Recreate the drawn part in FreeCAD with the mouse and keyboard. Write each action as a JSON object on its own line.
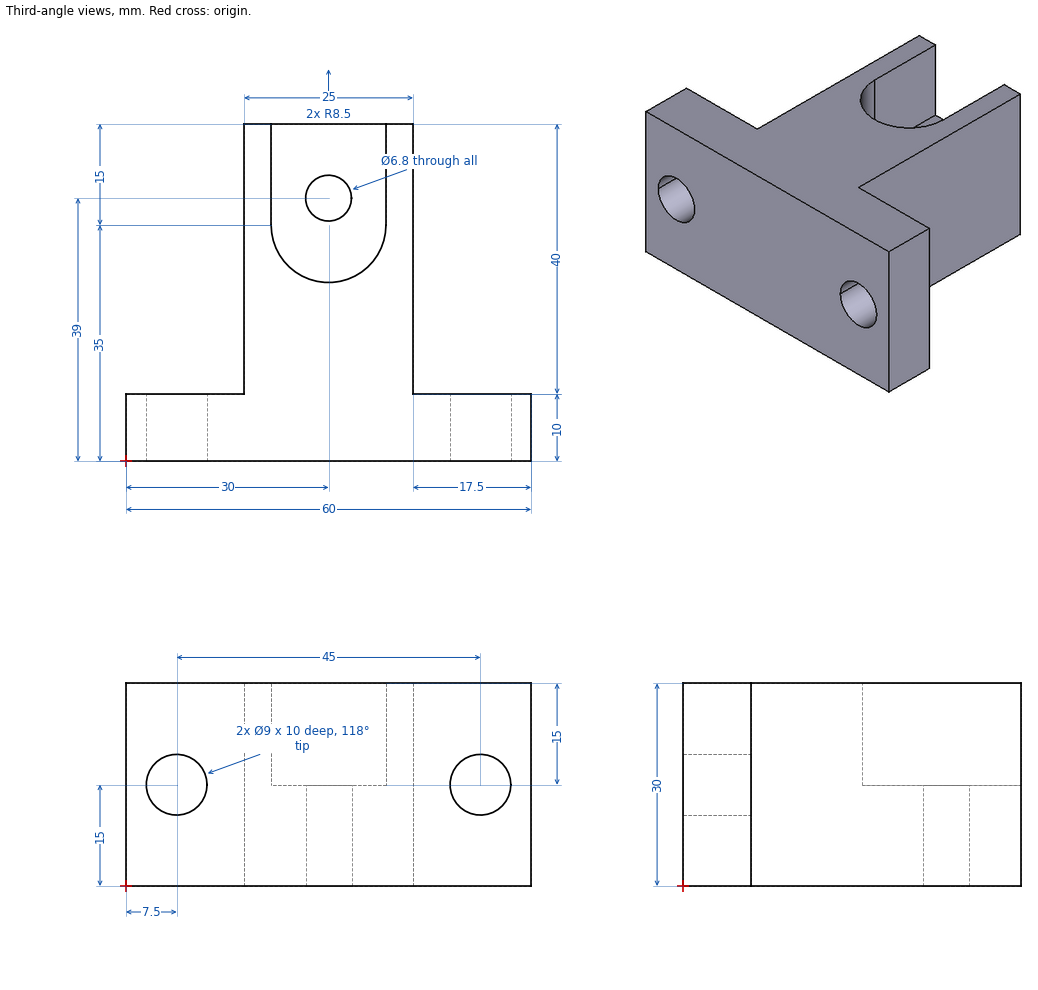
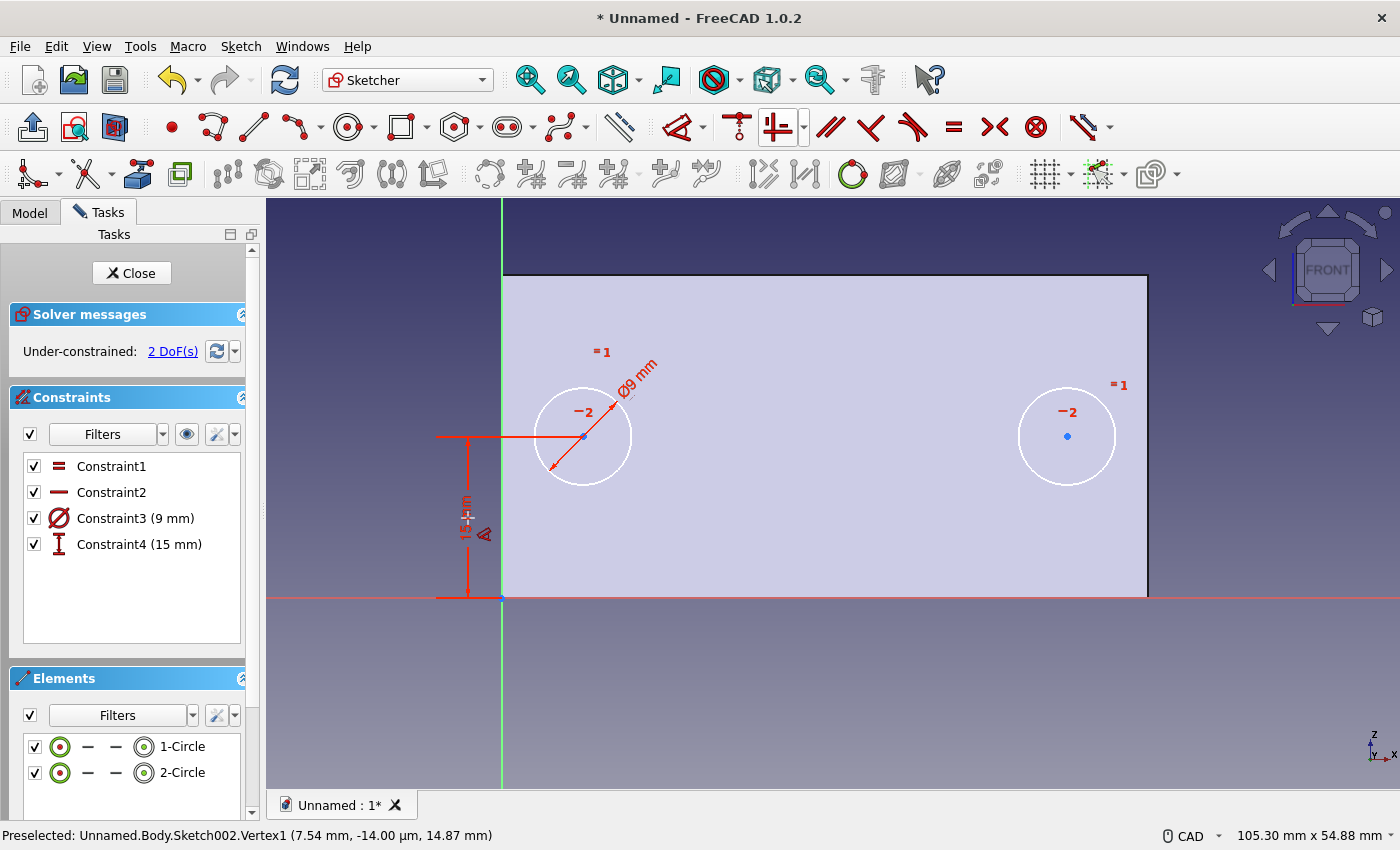
{"action": "left_click", "coordinate": [583, 437]}
{"action": "left_click", "coordinate": [542, 632]}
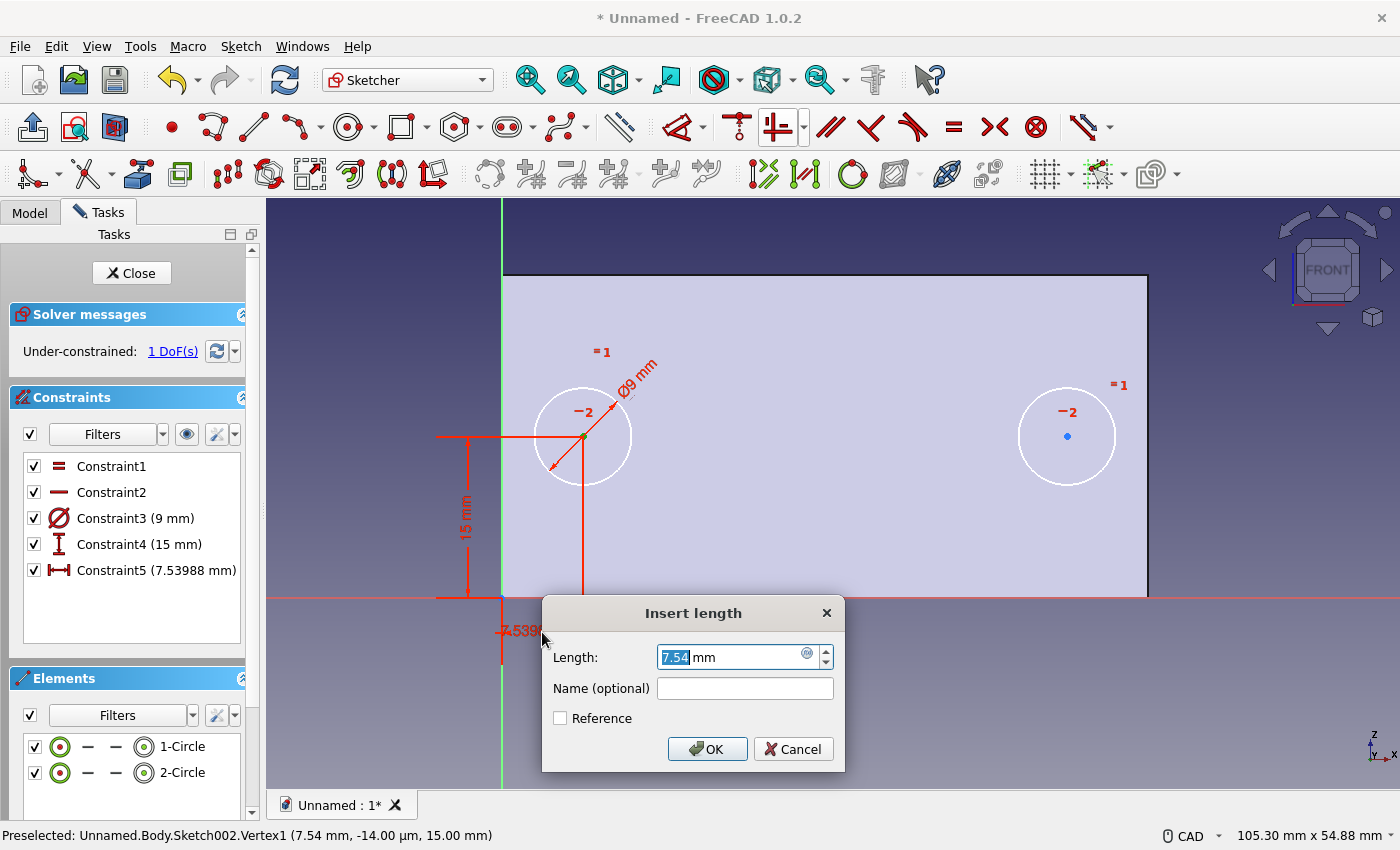
{"action": "type", "text": "7.5"}
{"action": "key", "text": "Return"}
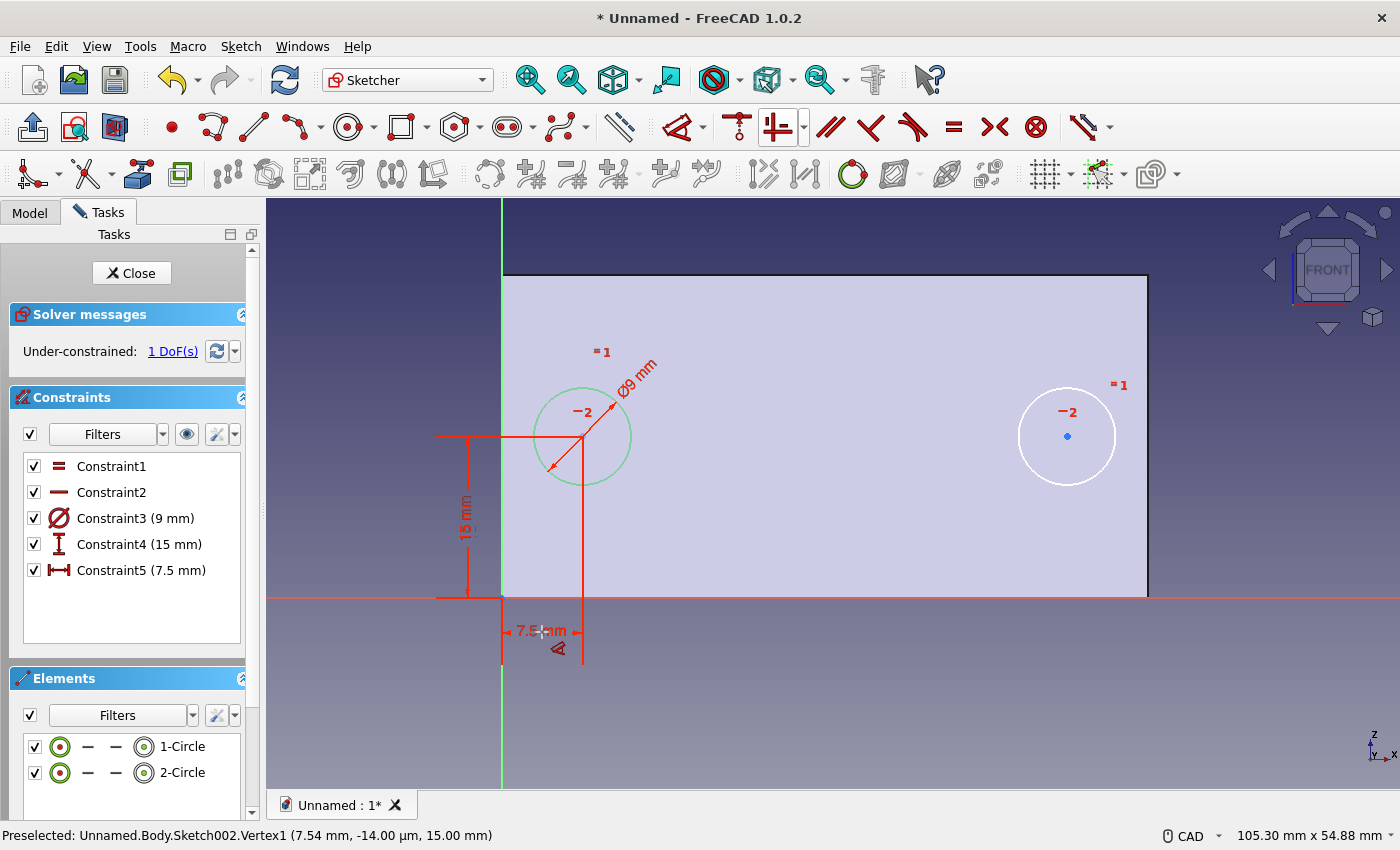
{"action": "left_click", "coordinate": [583, 437]}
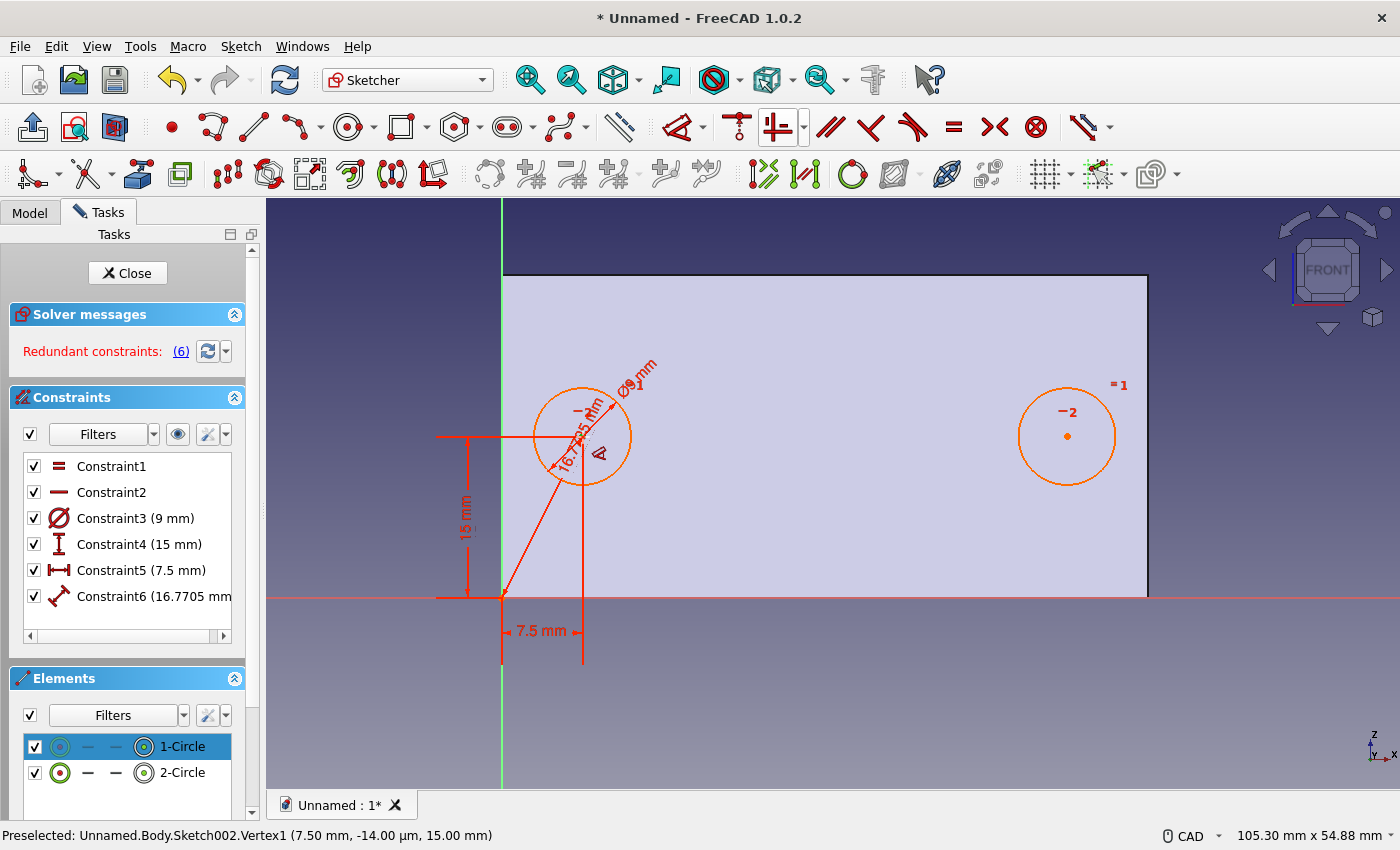
{"action": "left_click", "coordinate": [1067, 437]}
{"action": "left_click", "coordinate": [825, 403]}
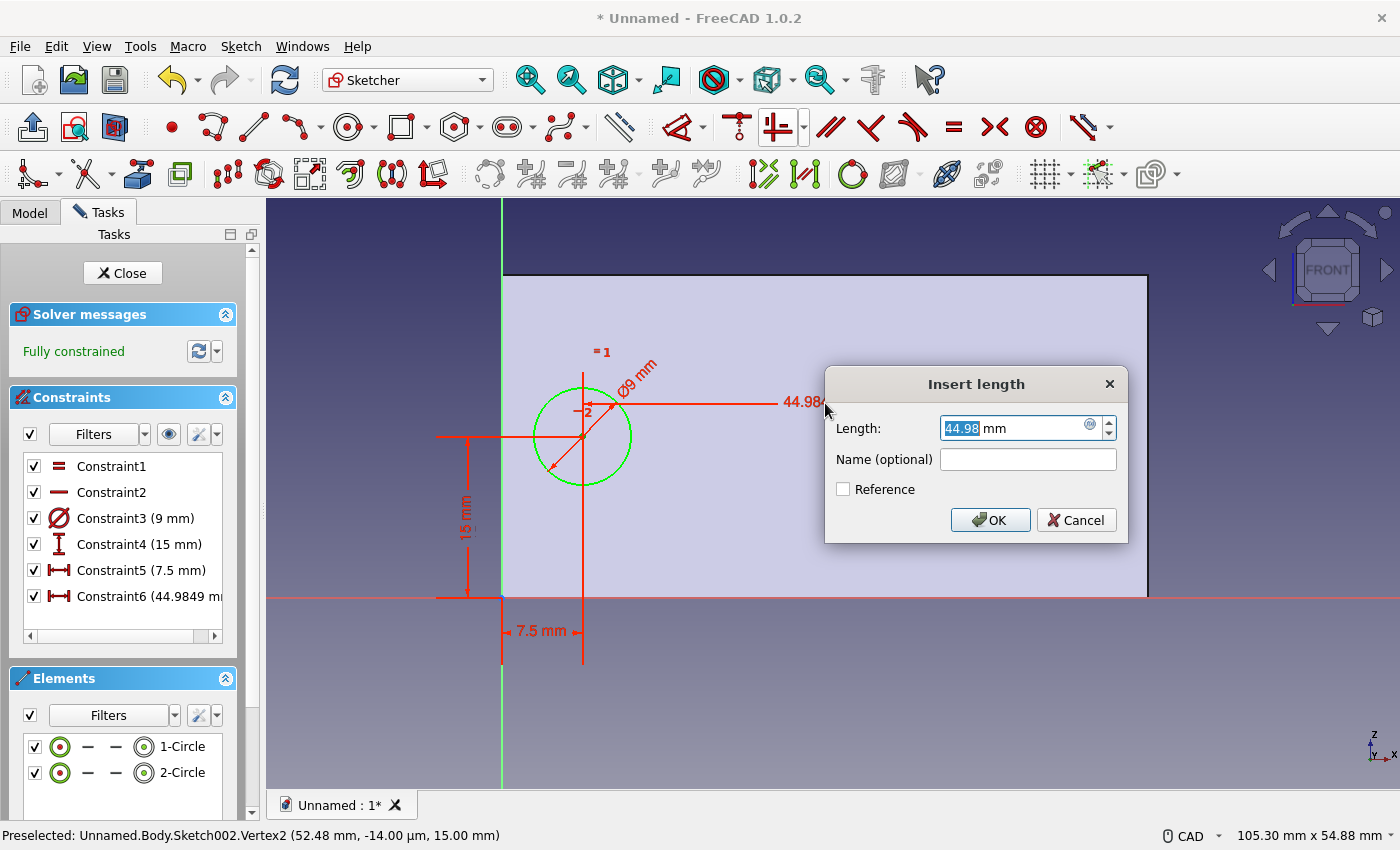
{"action": "type", "text": "45"}
{"action": "key", "text": "Return"}
{"action": "key", "text": "Escape"}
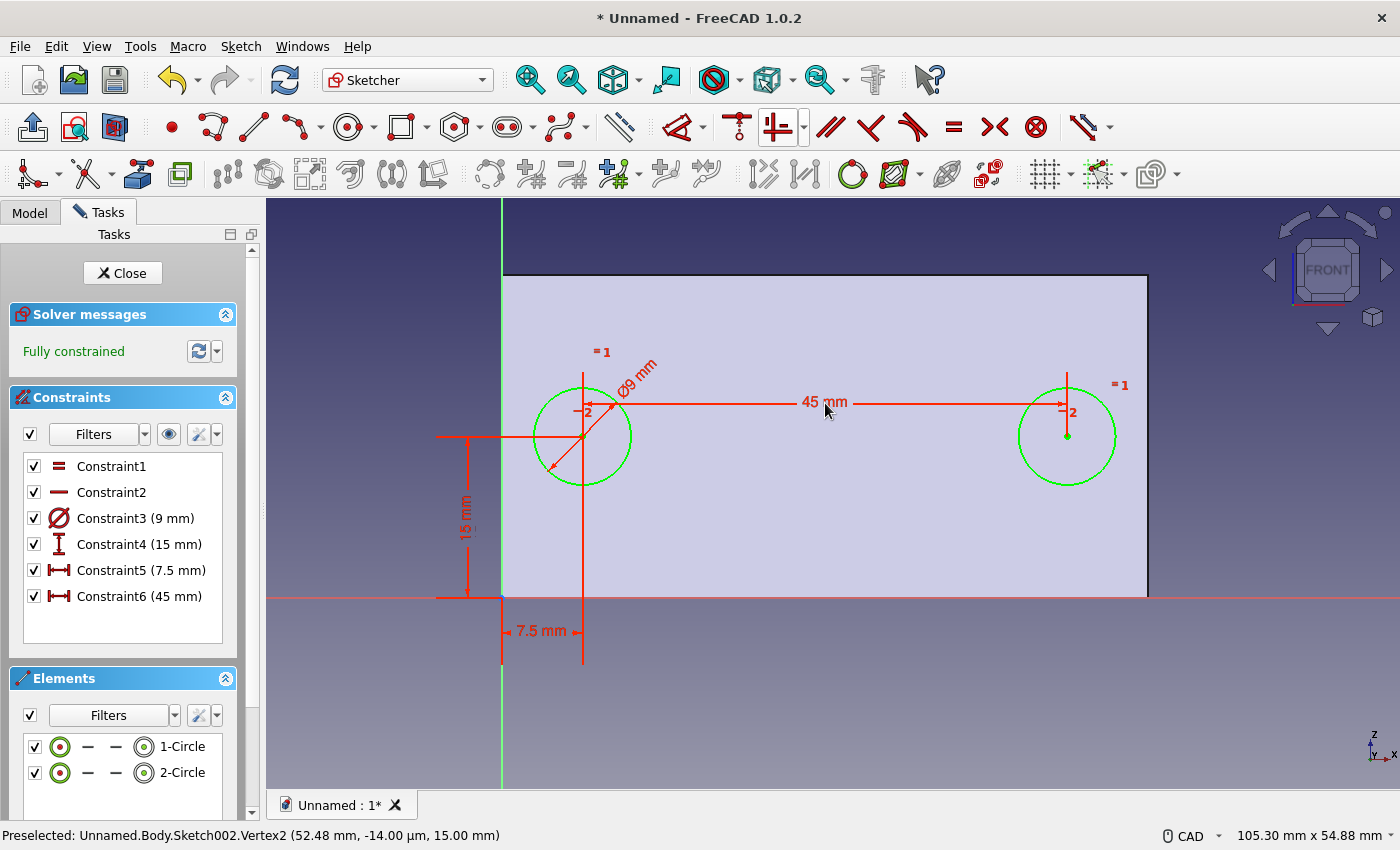
{"action": "left_click", "coordinate": [123, 273]}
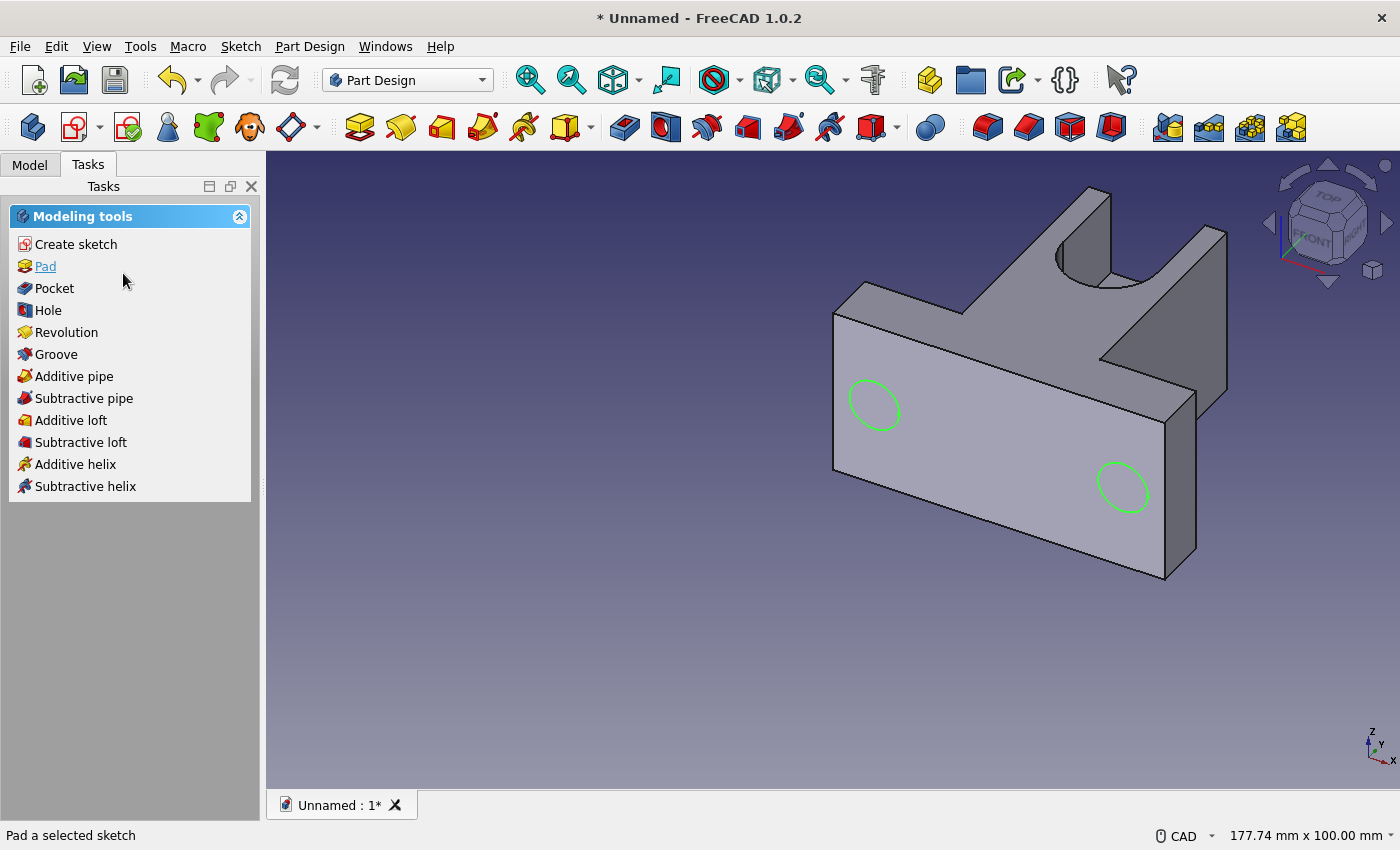
{"action": "left_click", "coordinate": [666, 128]}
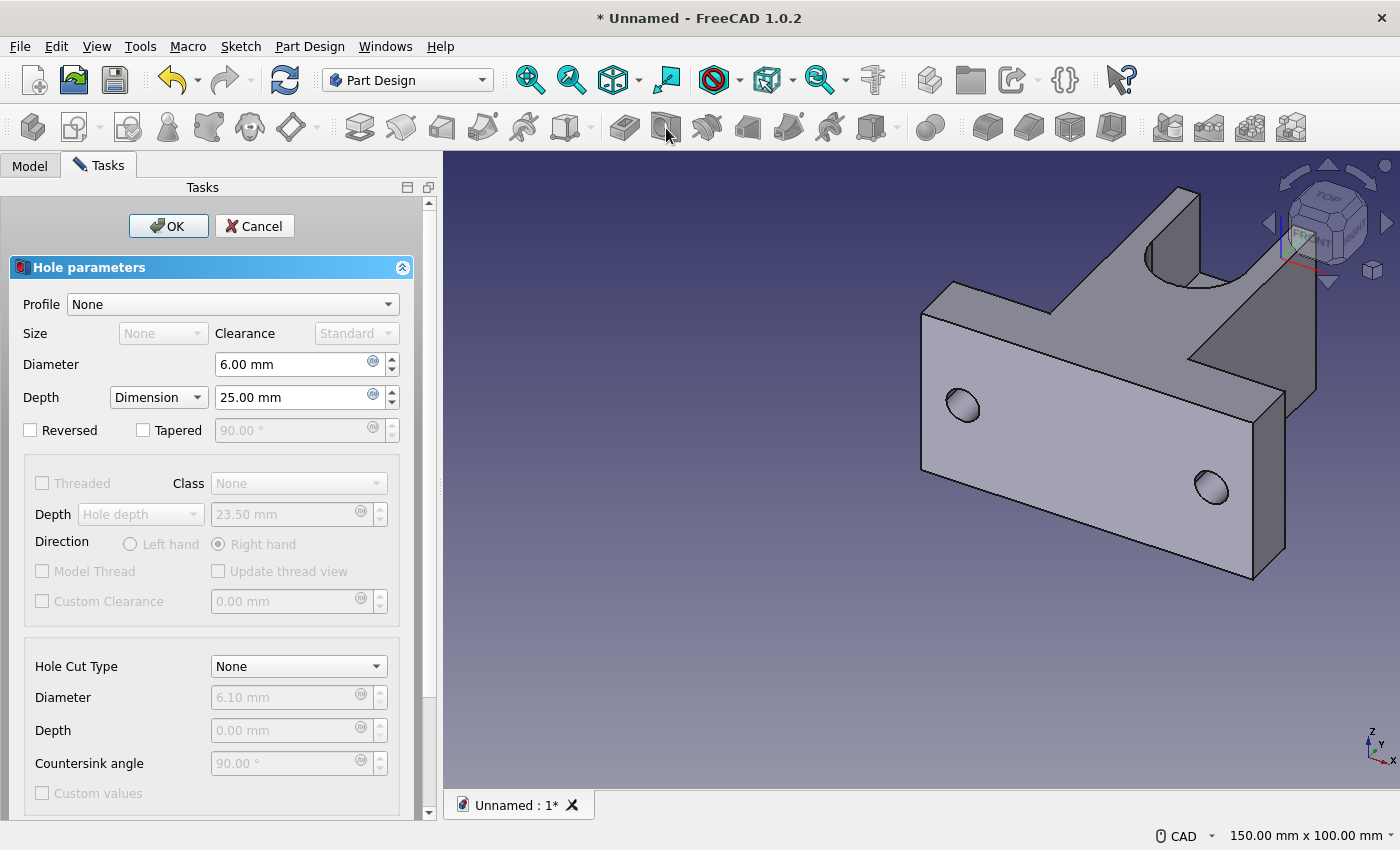
{"action": "triple_click", "coordinate": [300, 364]}